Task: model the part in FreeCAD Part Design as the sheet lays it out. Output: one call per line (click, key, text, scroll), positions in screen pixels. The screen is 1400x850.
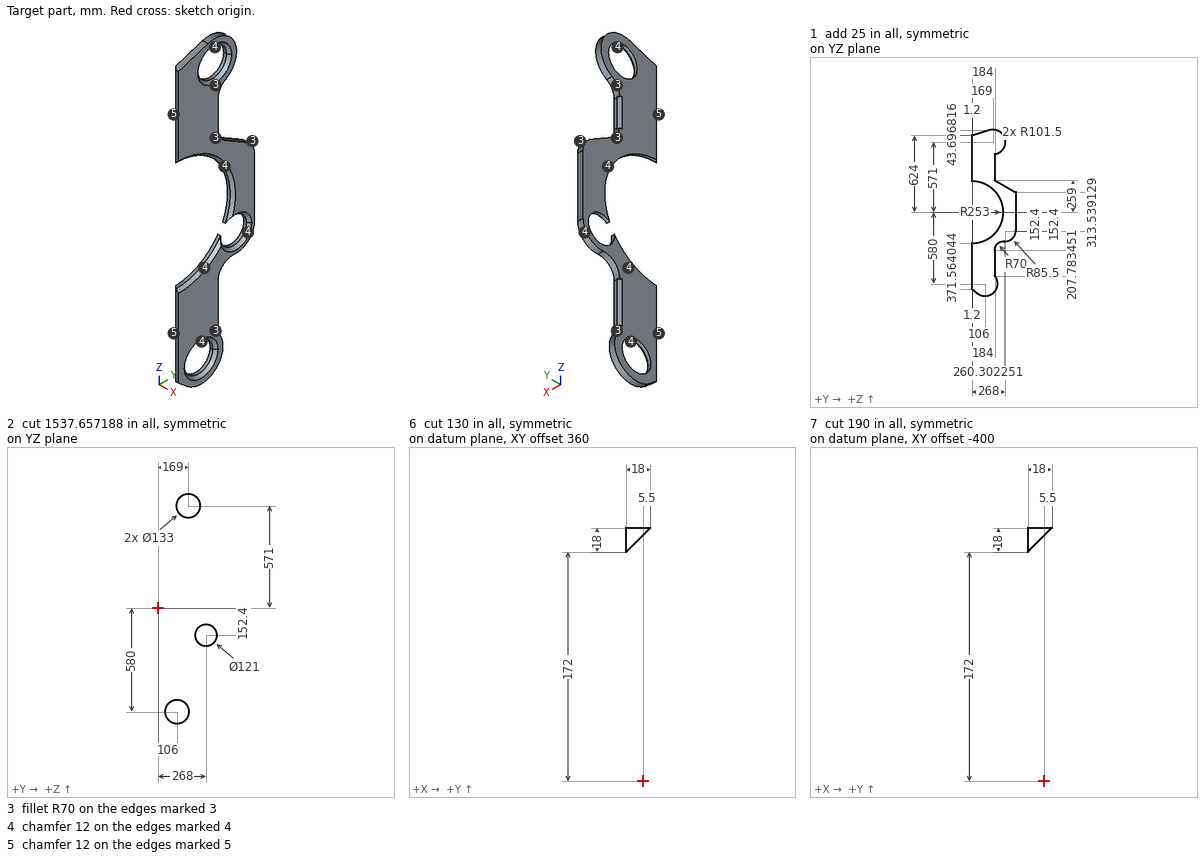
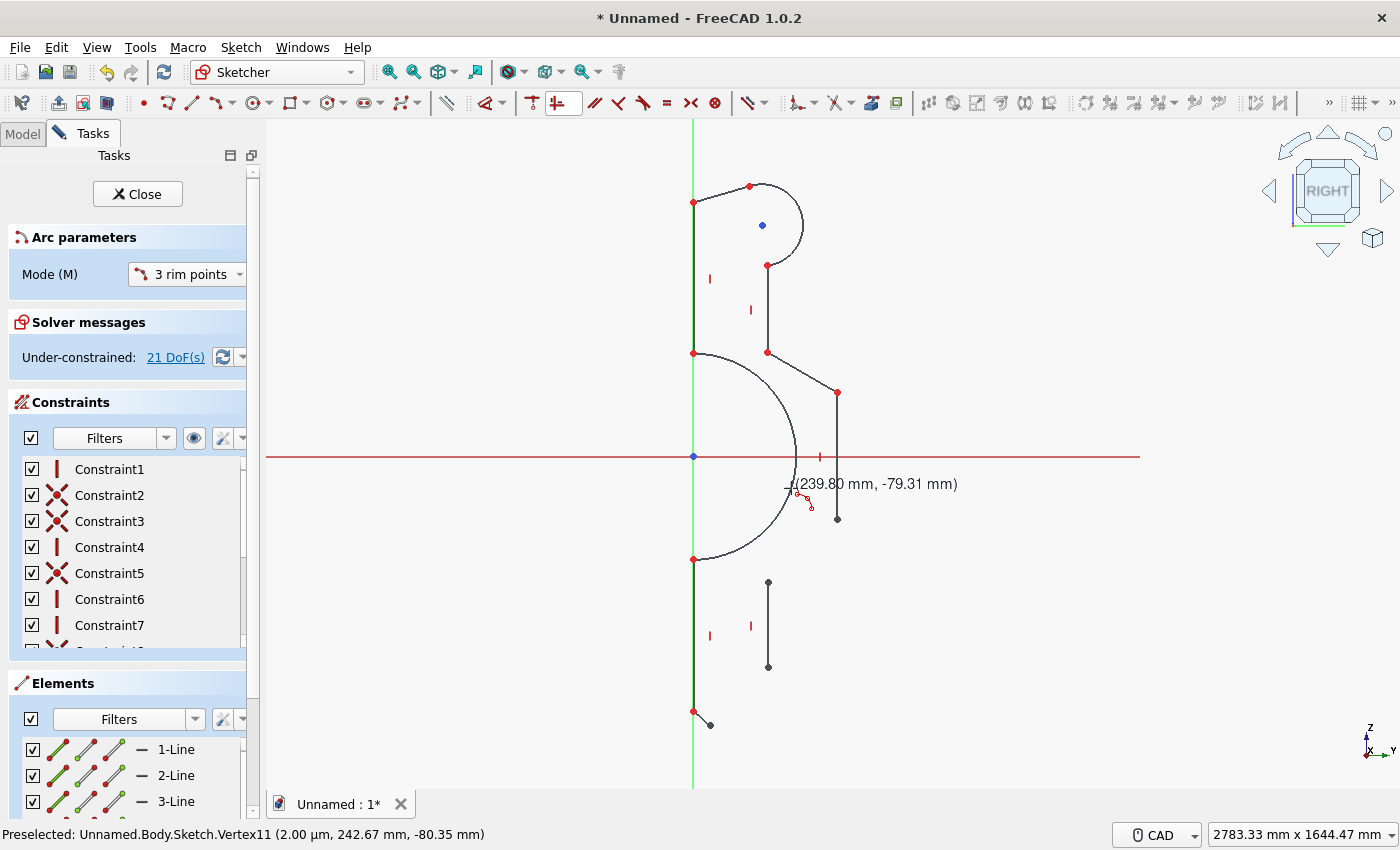
scroll(710, 725, up, 3)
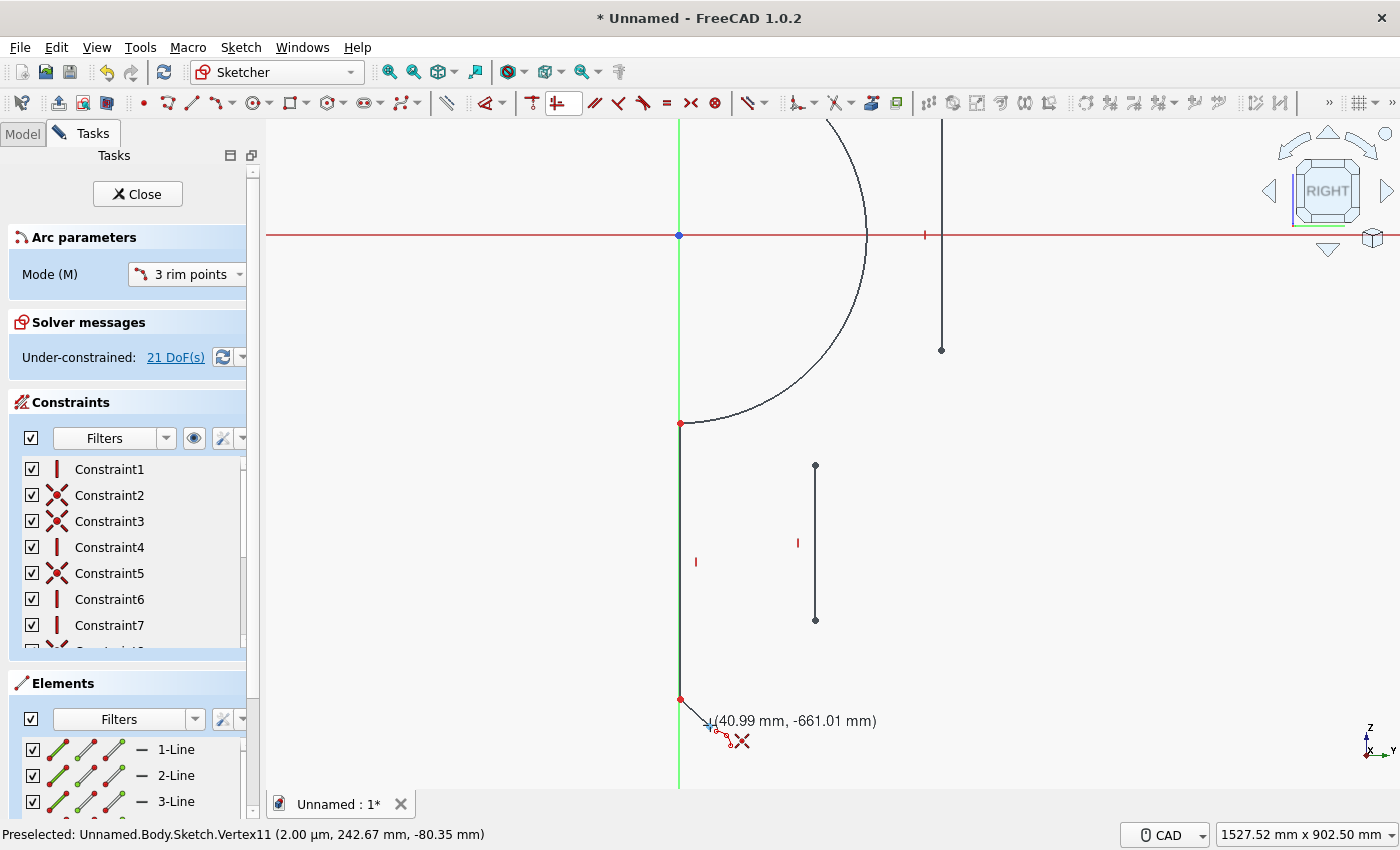
click(710, 726)
click(815, 620)
click(811, 719)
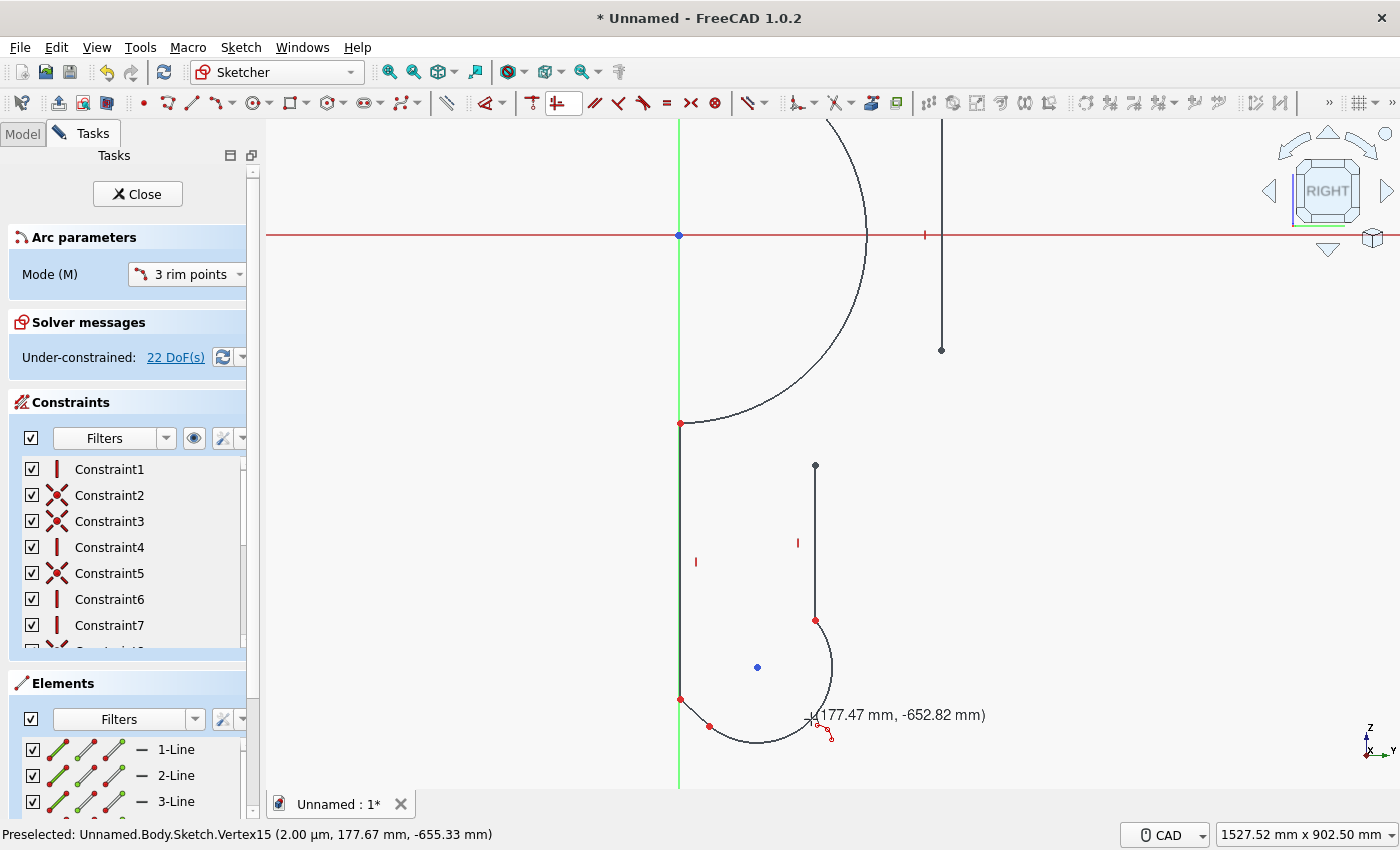
click(815, 466)
click(872, 412)
click(833, 425)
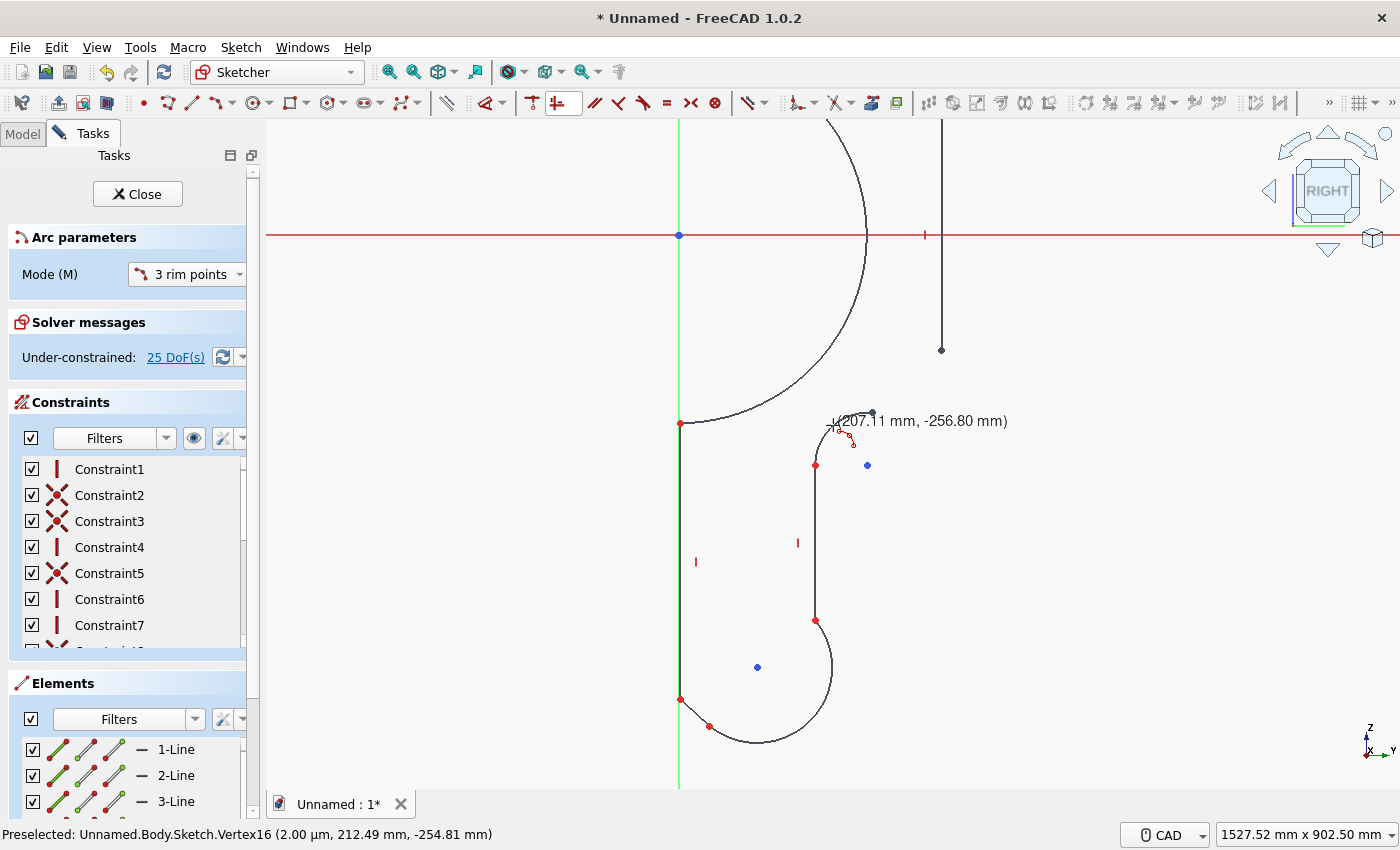
click(872, 413)
click(942, 350)
click(921, 395)
key(Escape)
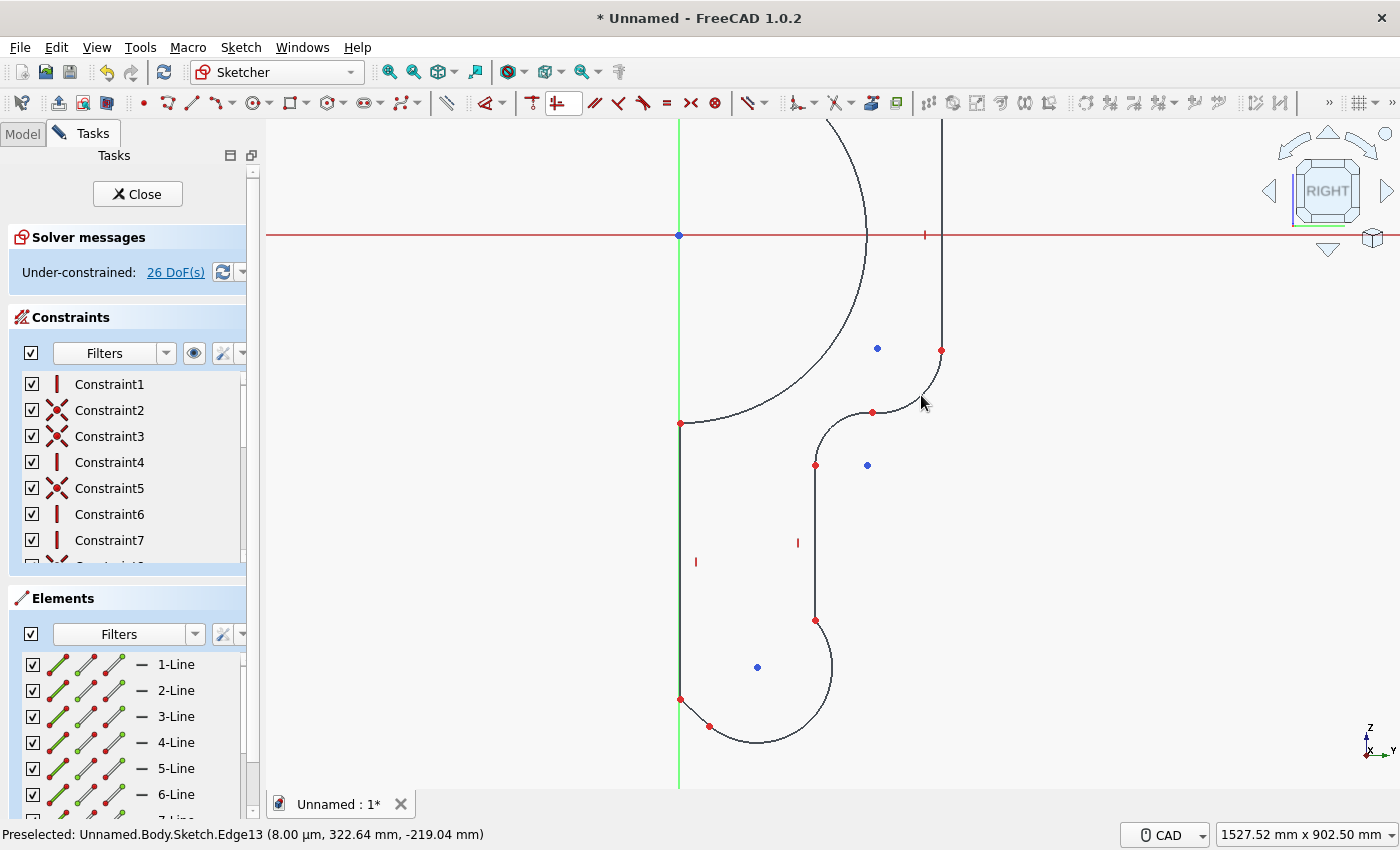
scroll(689, 707, up, 2)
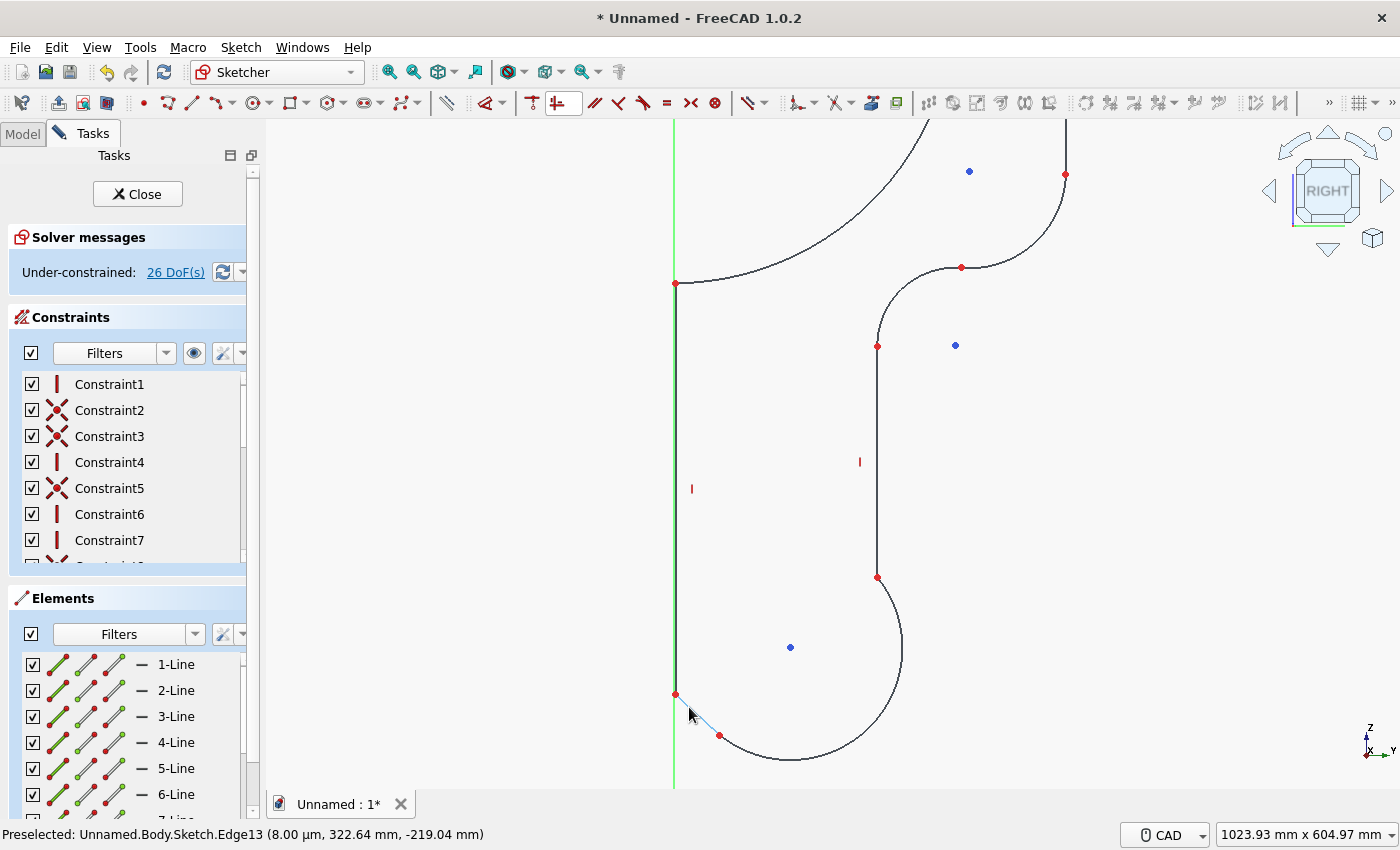
click(689, 707)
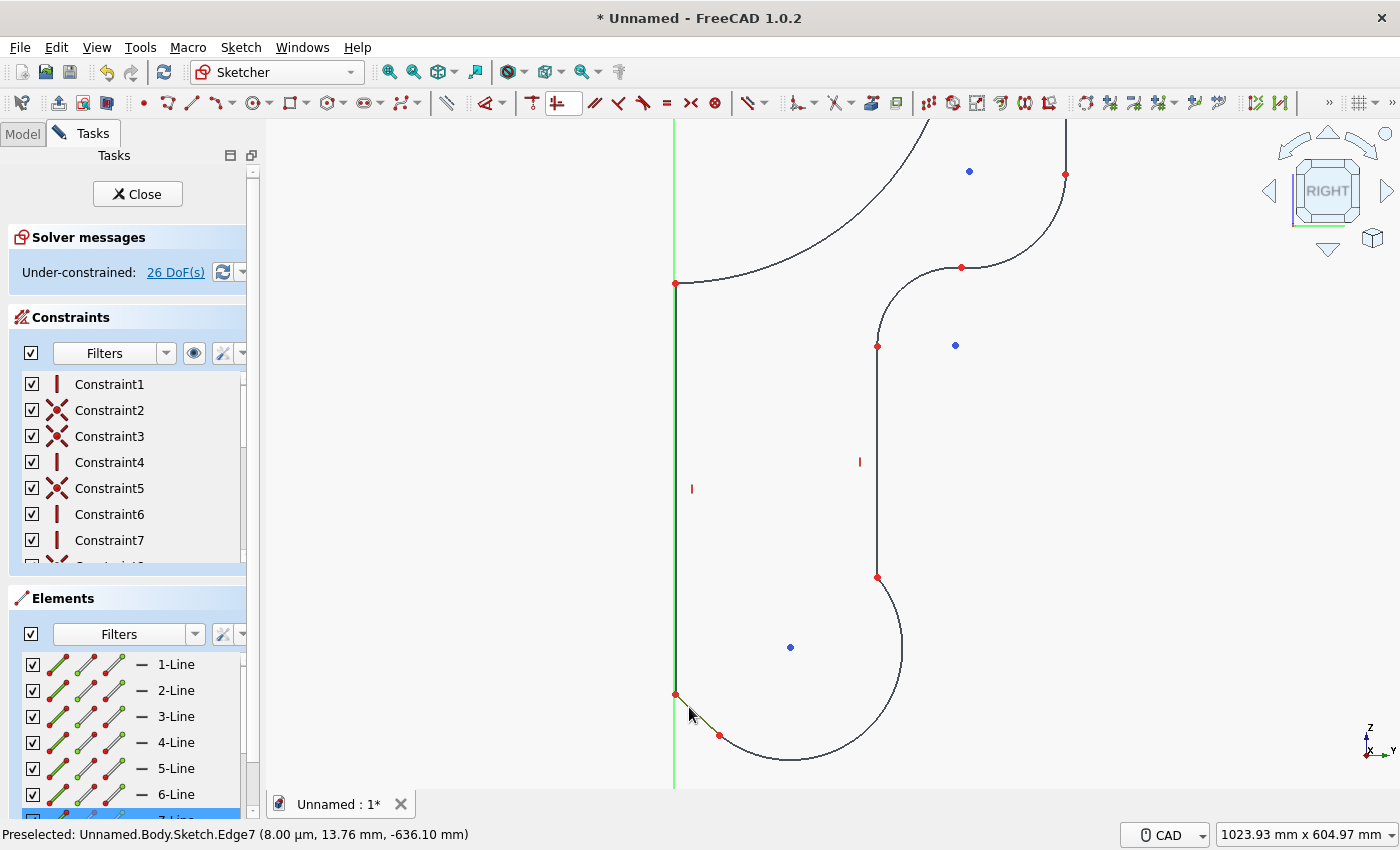
click(812, 758)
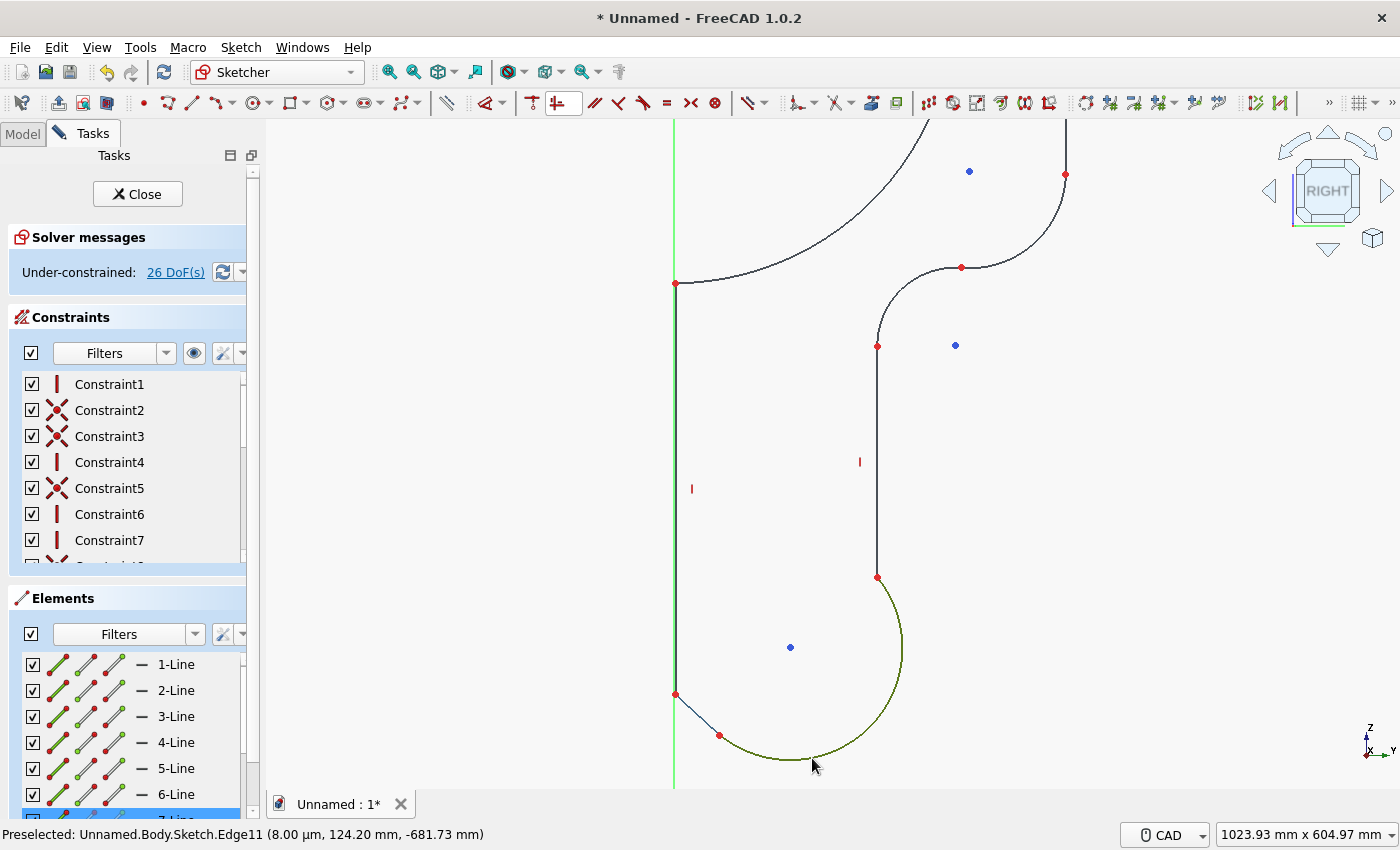
click(644, 104)